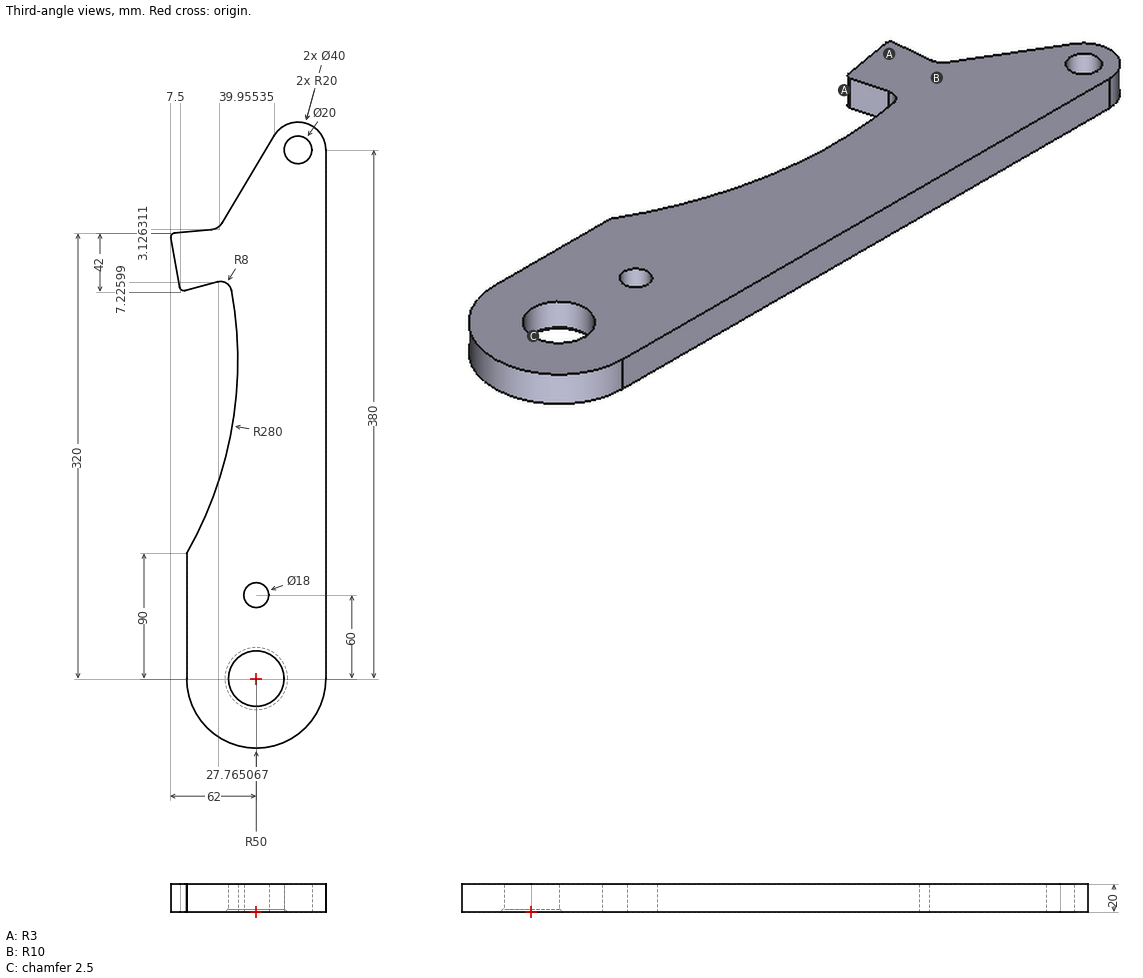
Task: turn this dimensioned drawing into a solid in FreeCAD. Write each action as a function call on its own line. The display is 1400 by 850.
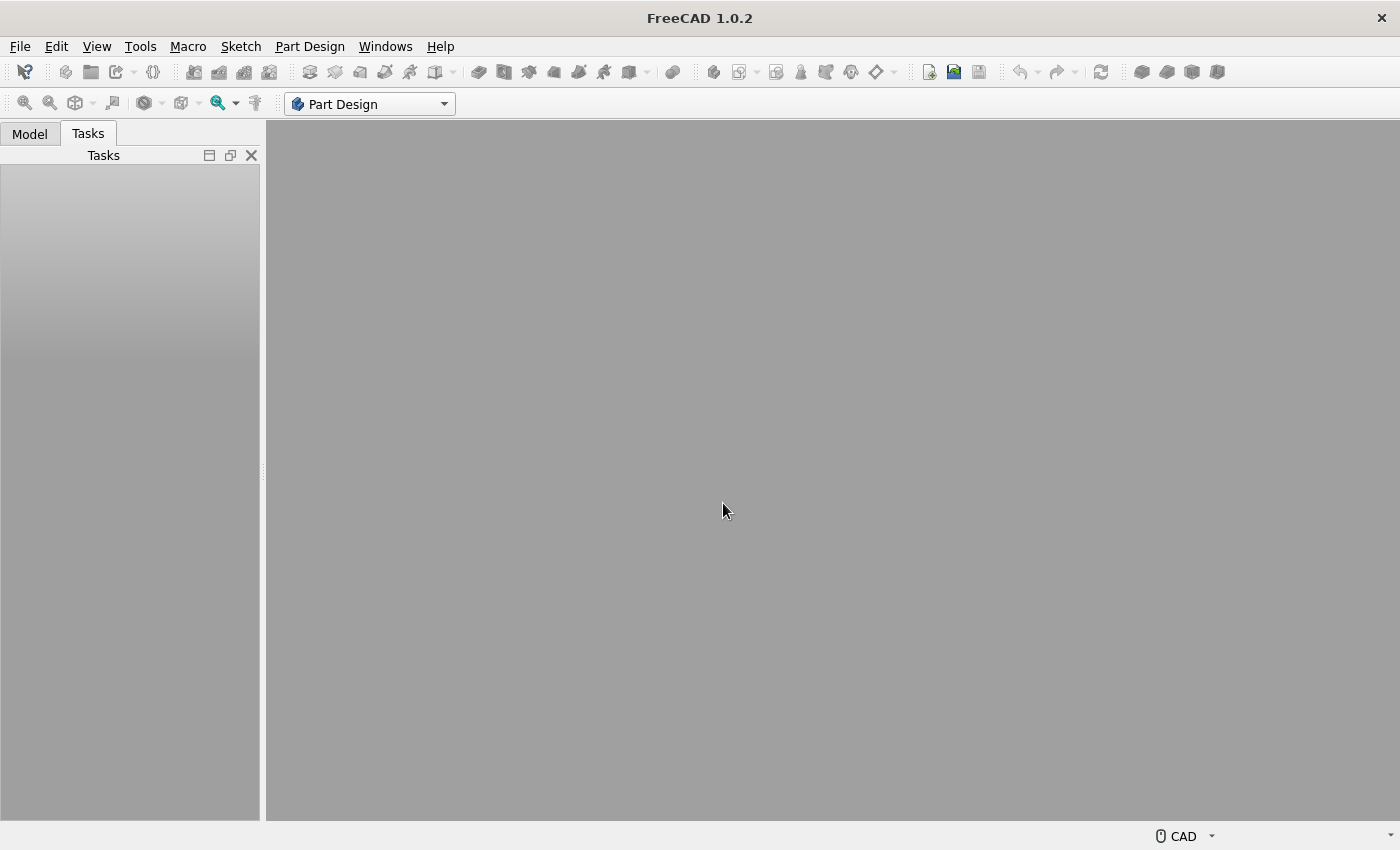
click(929, 72)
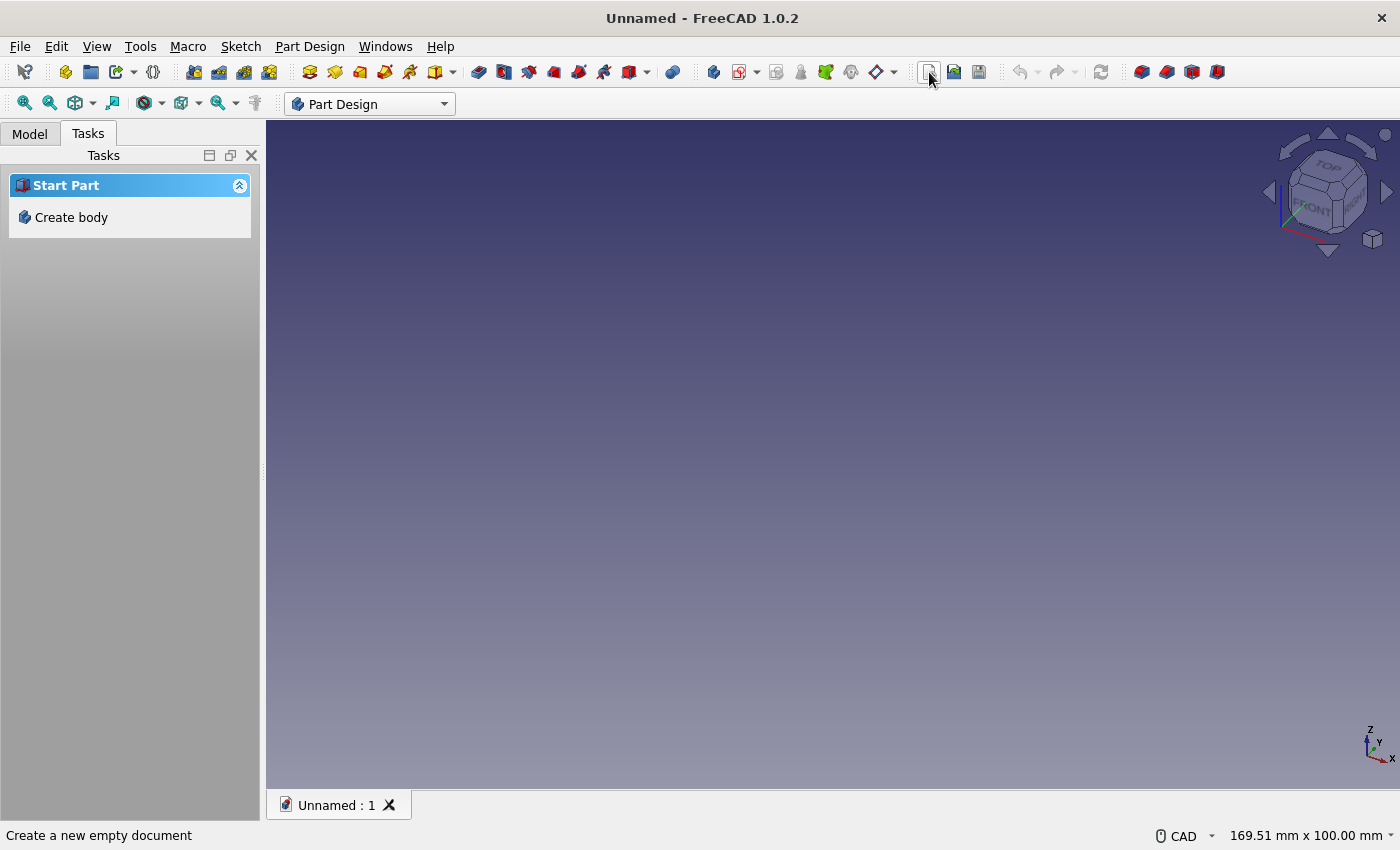
click(738, 72)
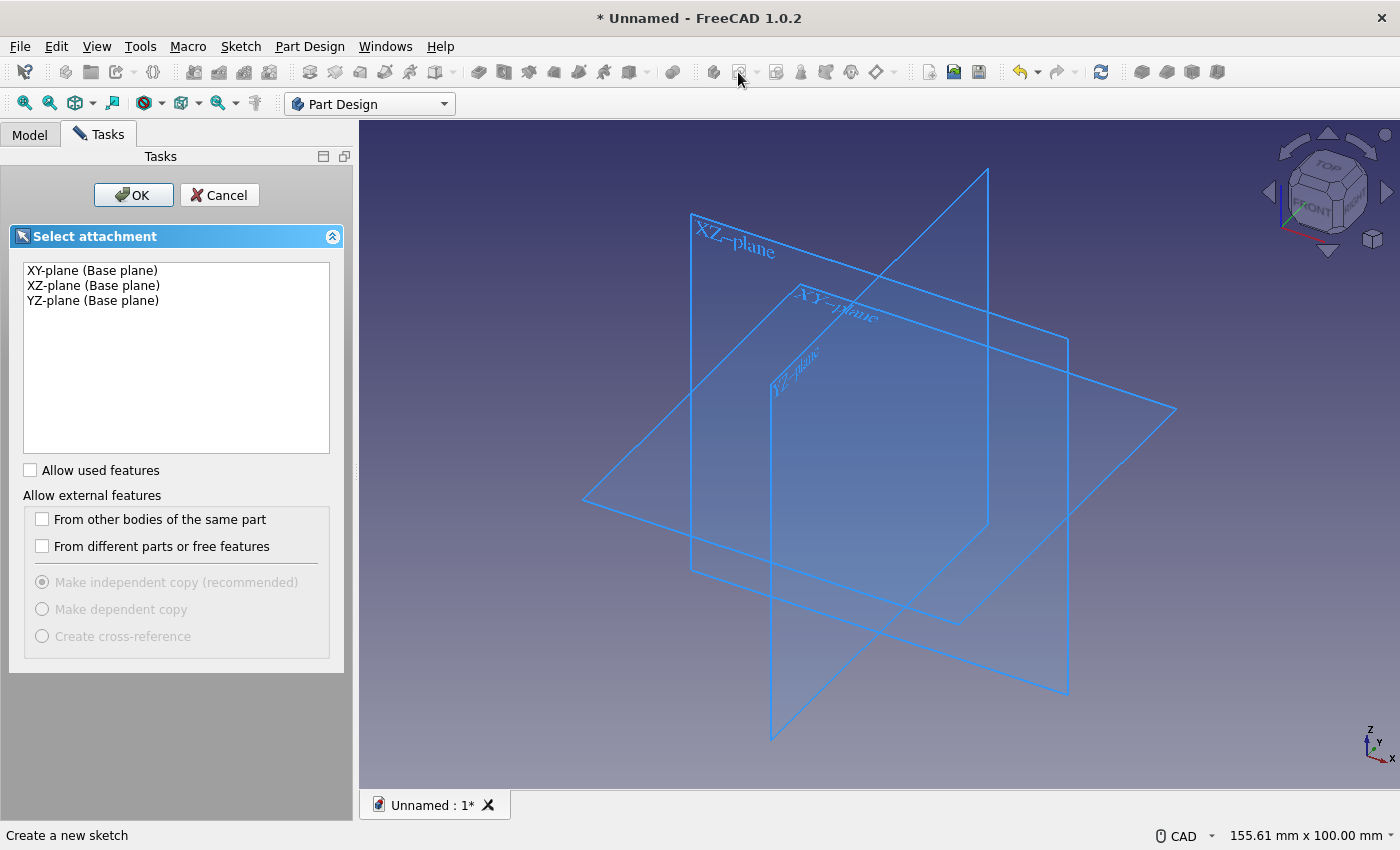
click(84, 270)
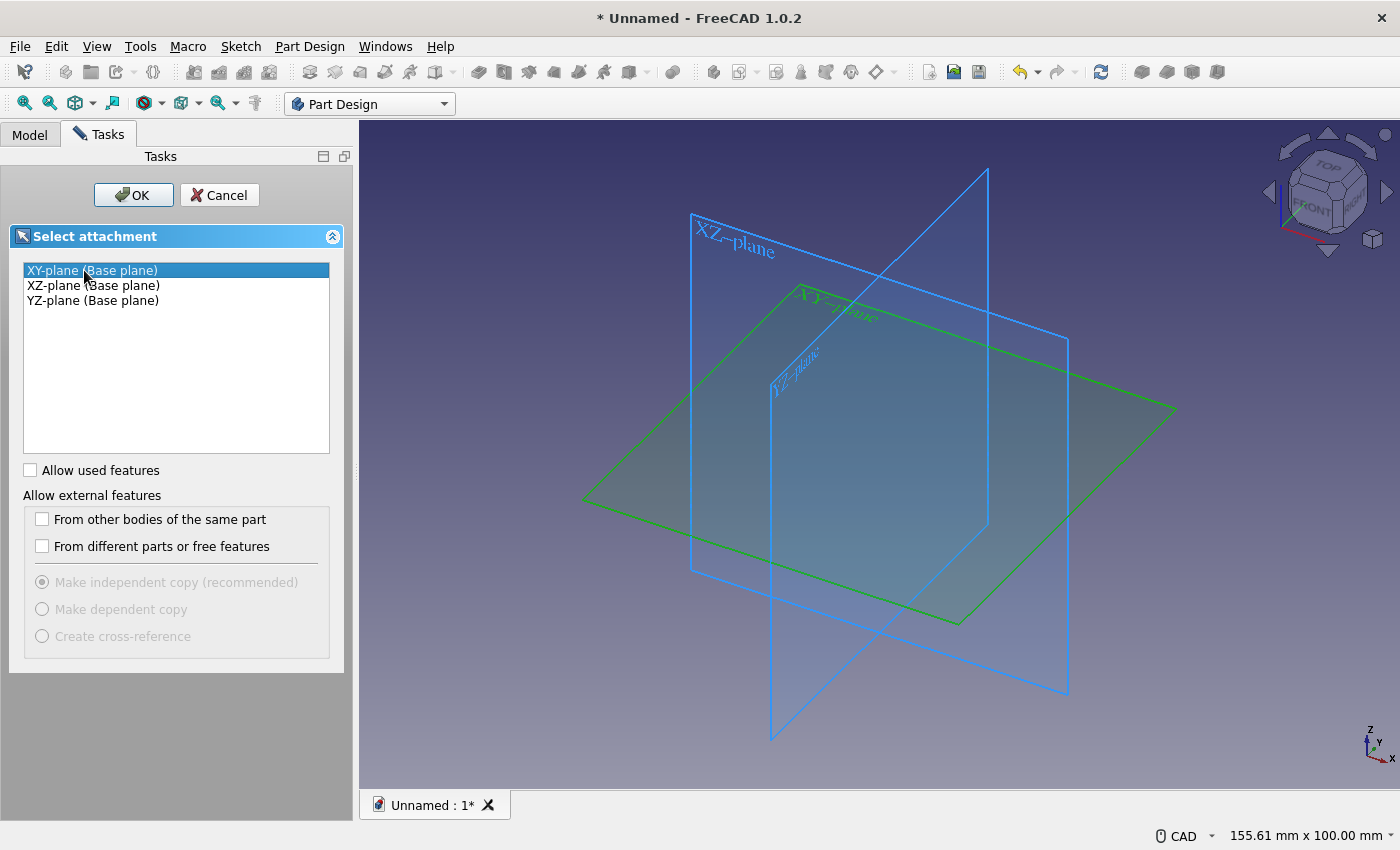
click(134, 195)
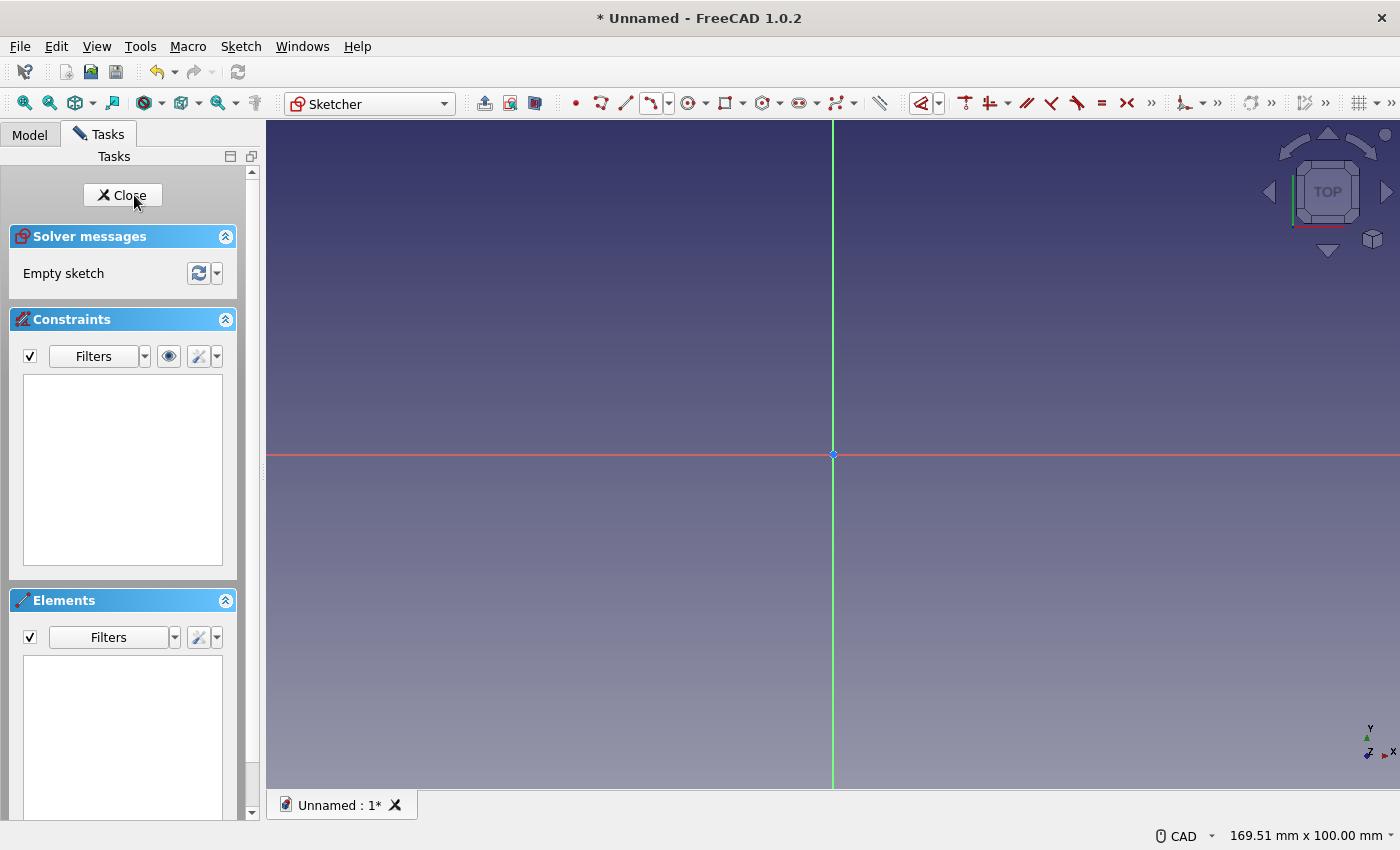
scroll(760, 637, down, 10)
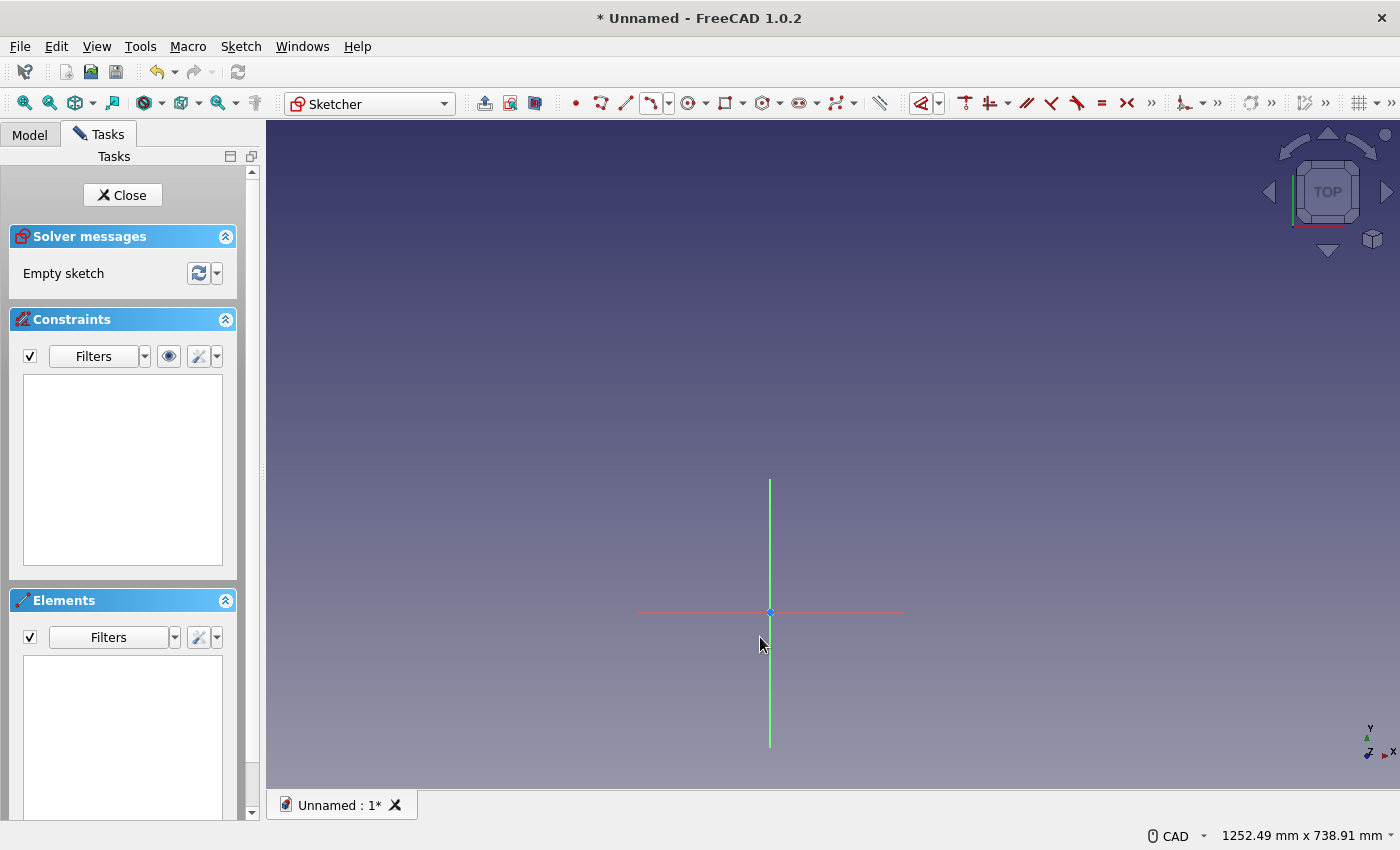
click(626, 104)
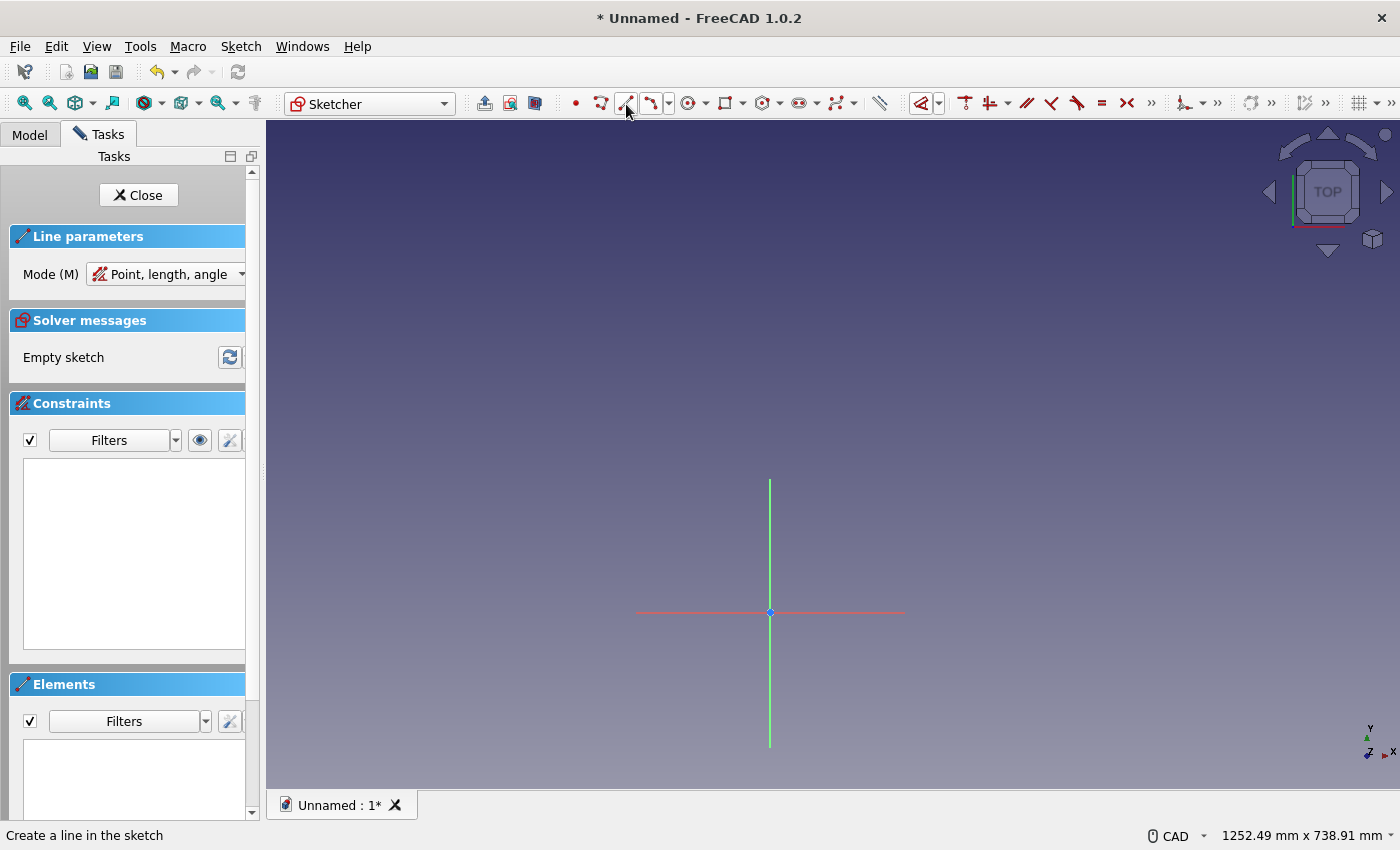
click(725, 531)
click(725, 613)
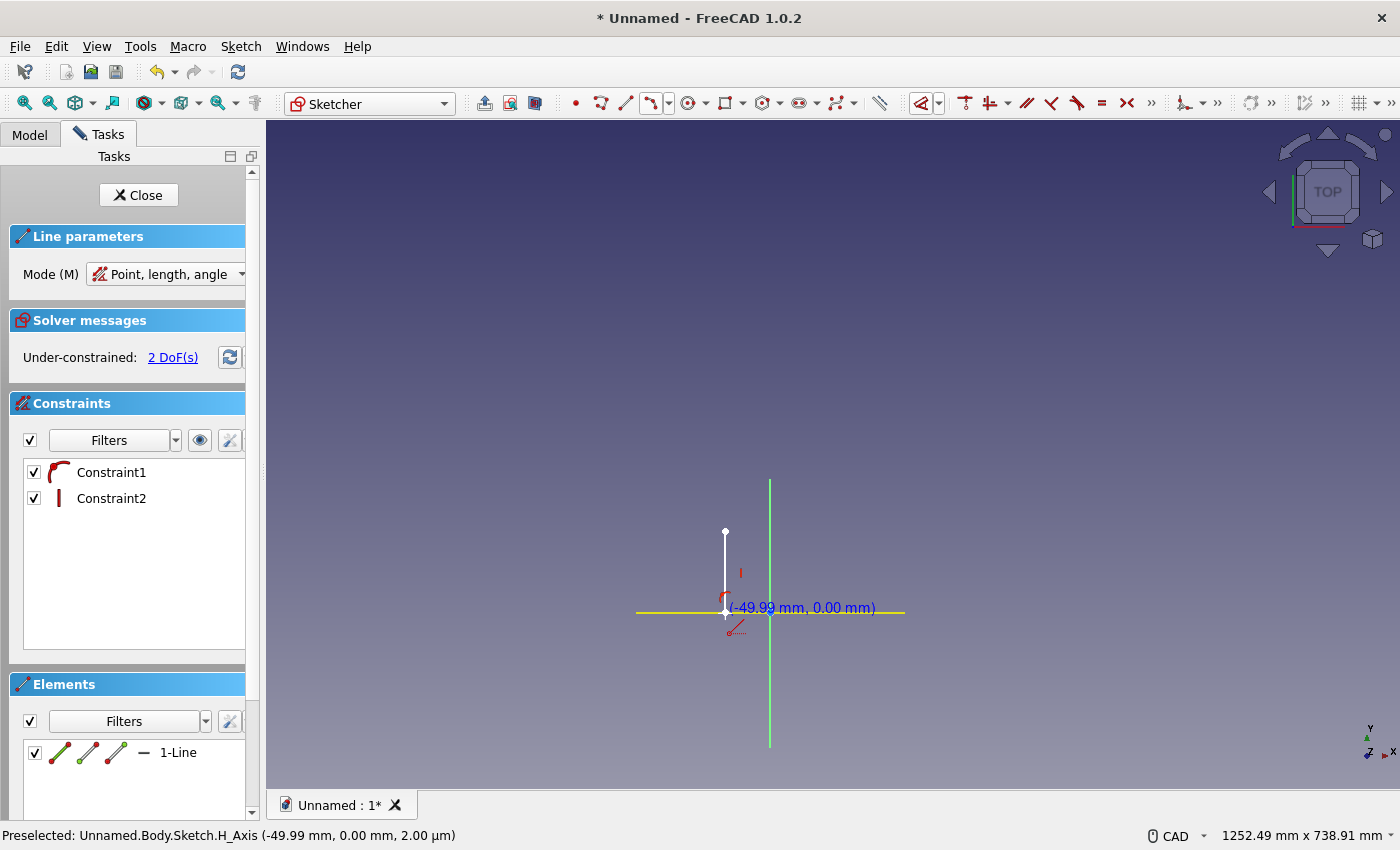
click(816, 613)
click(816, 269)